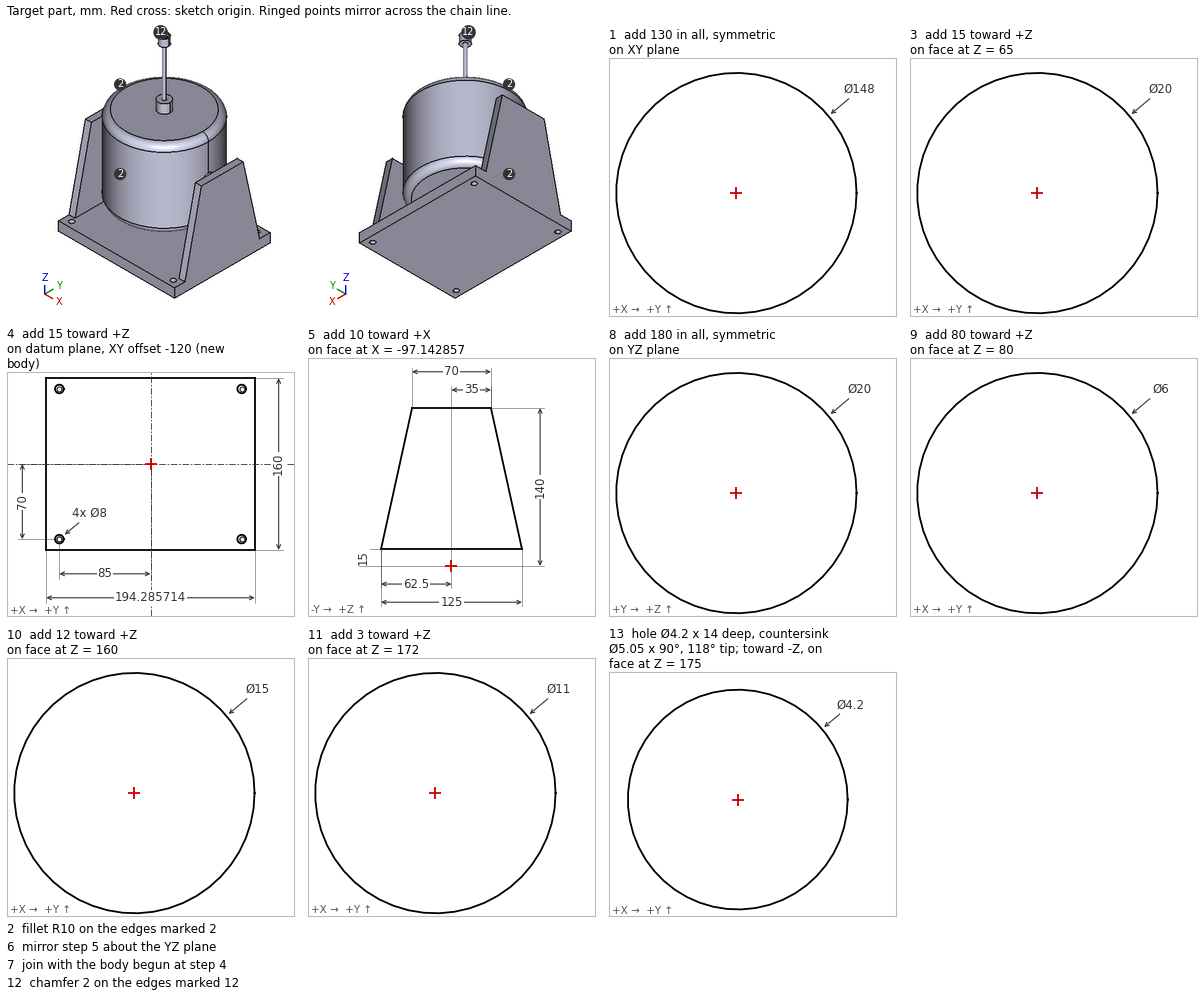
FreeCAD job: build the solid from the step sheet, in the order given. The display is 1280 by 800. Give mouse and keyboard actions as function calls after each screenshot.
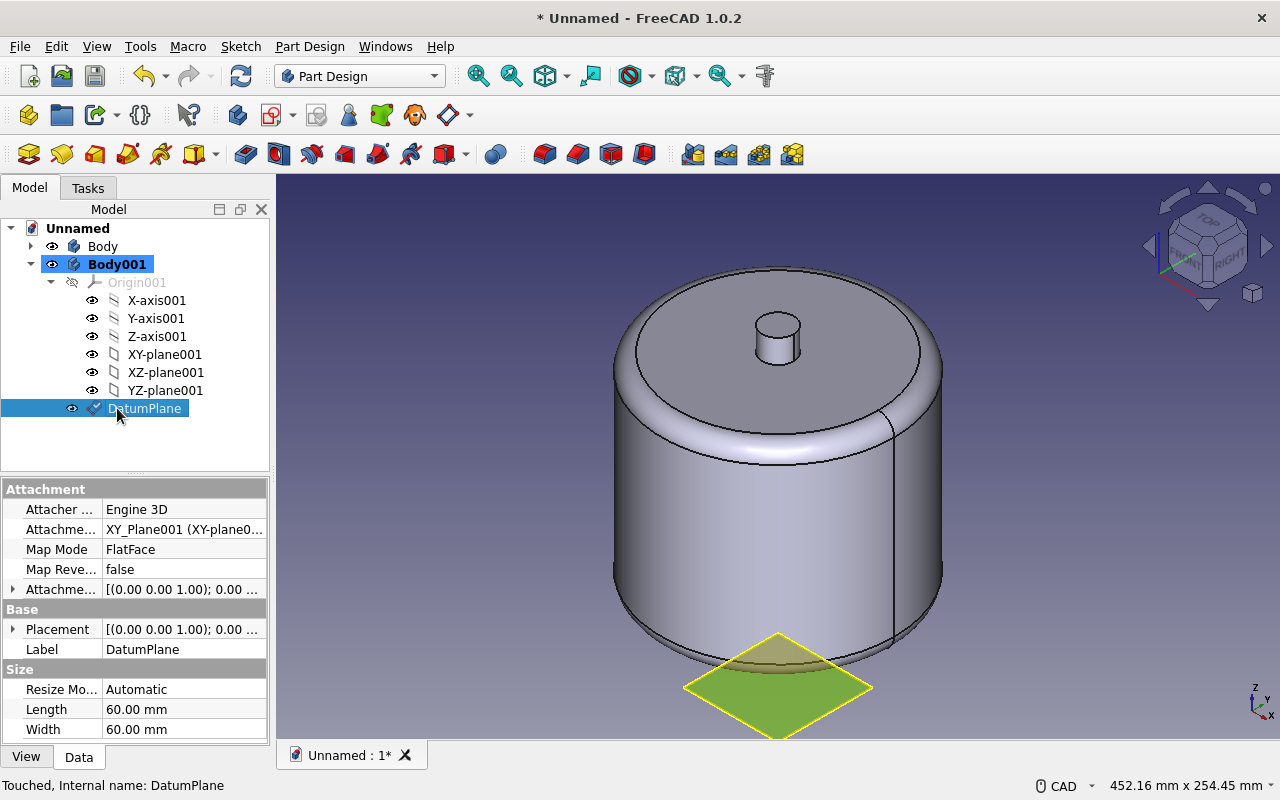
click(270, 116)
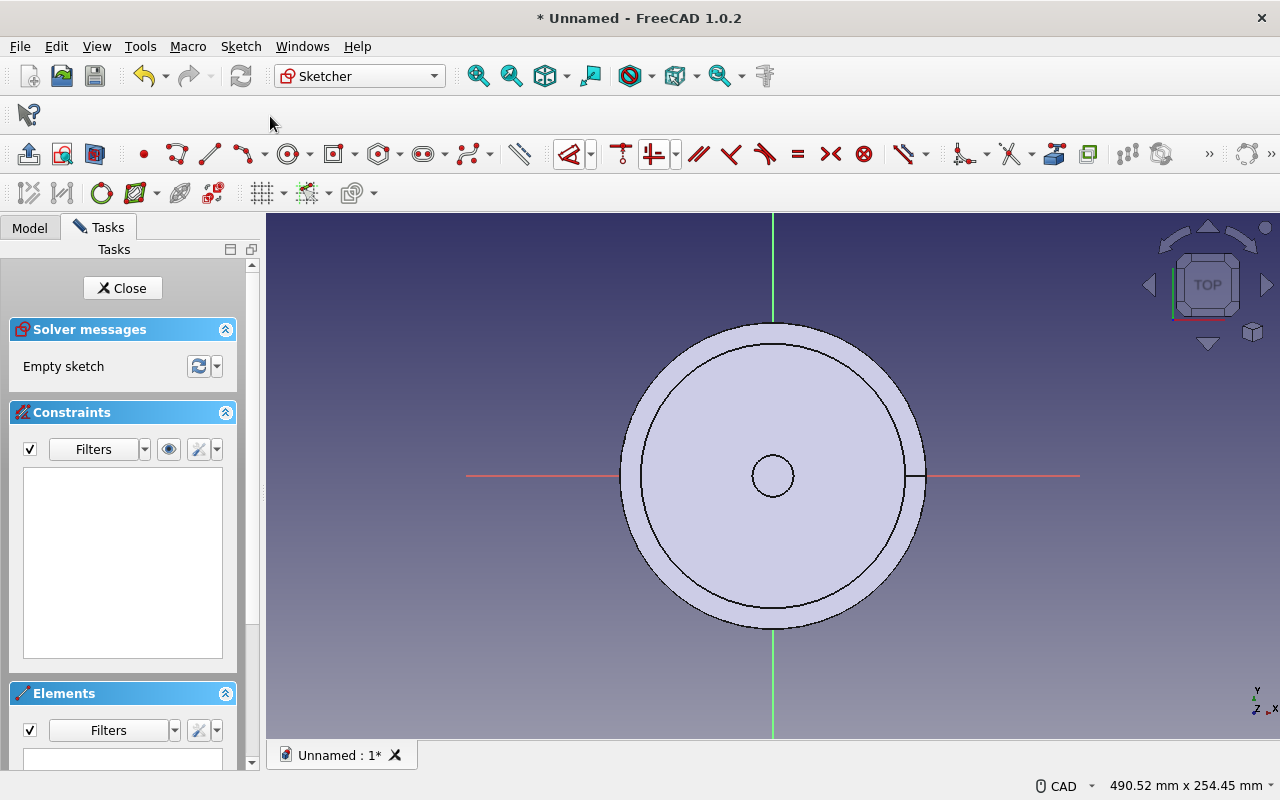
key(g)
key(v)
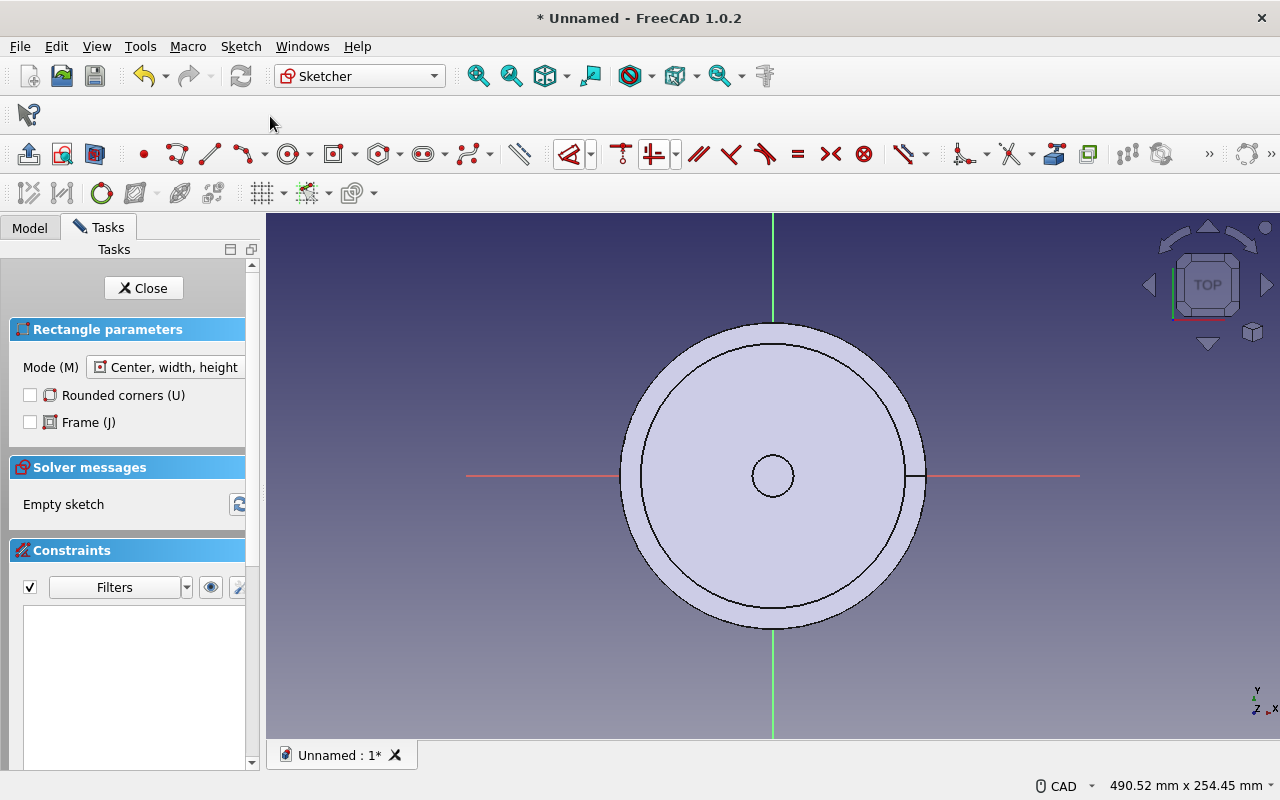
click(773, 476)
click(974, 311)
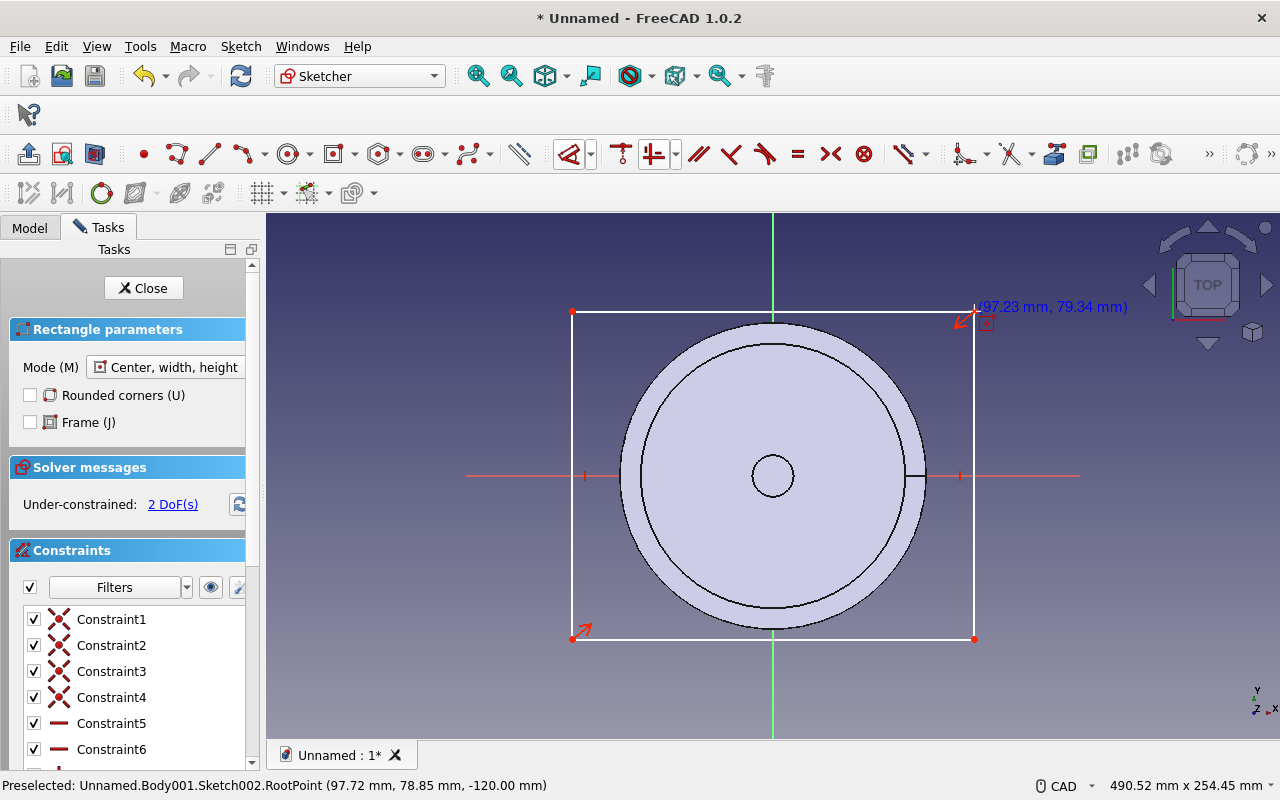
key(g)
key(c)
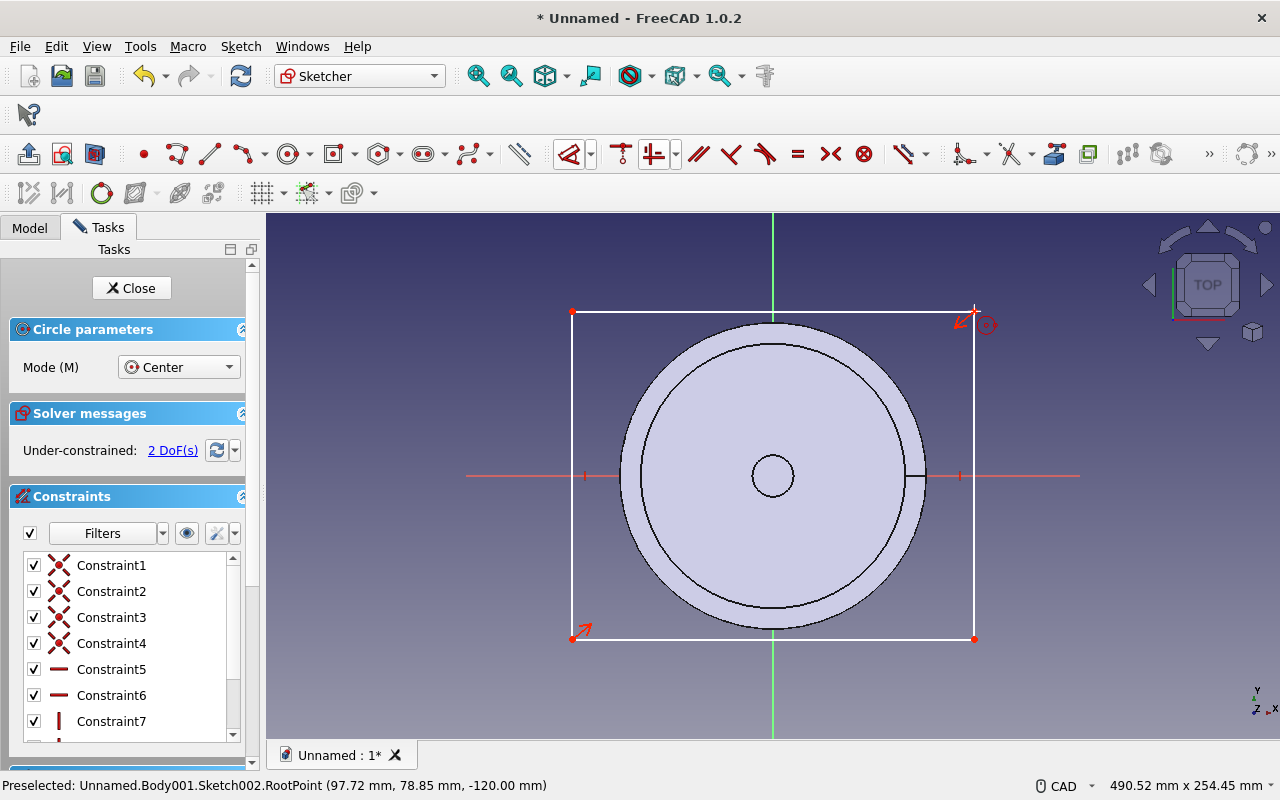
scroll(597, 621, up, 6)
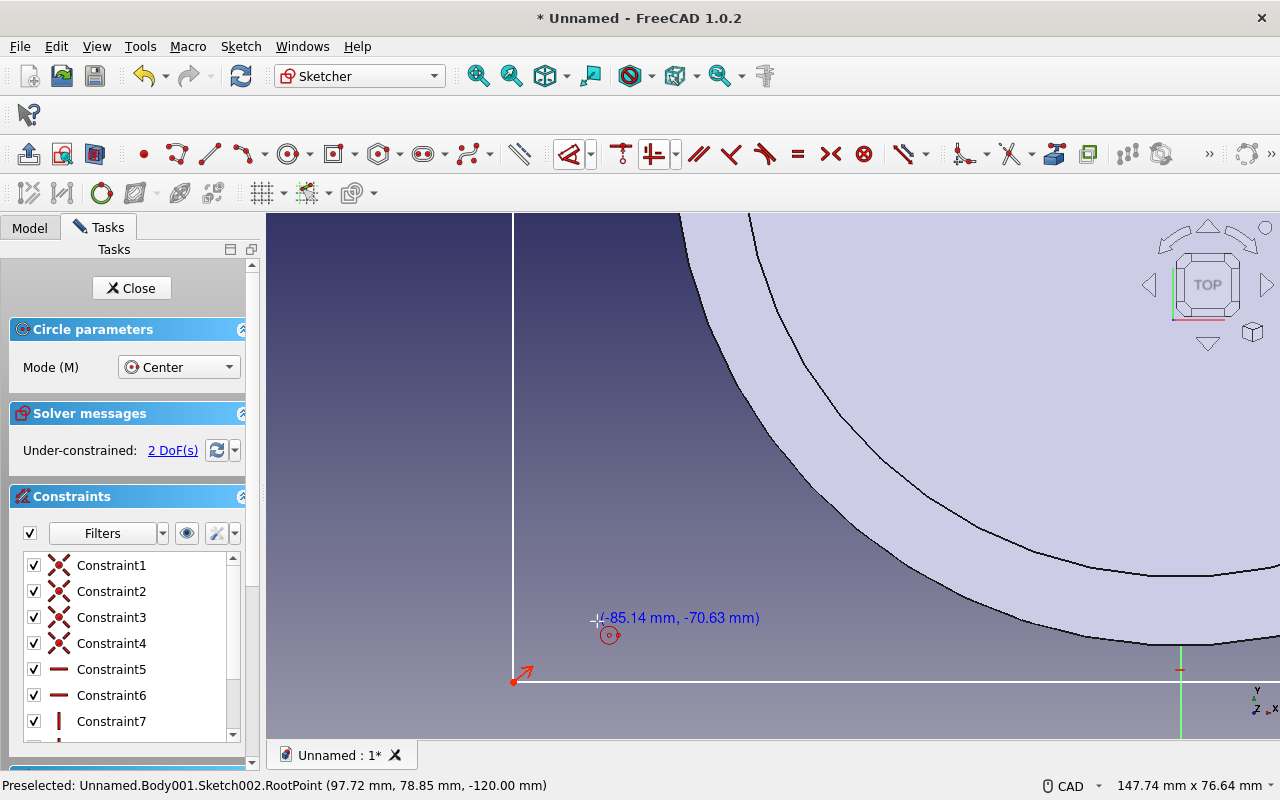
click(597, 618)
click(617, 599)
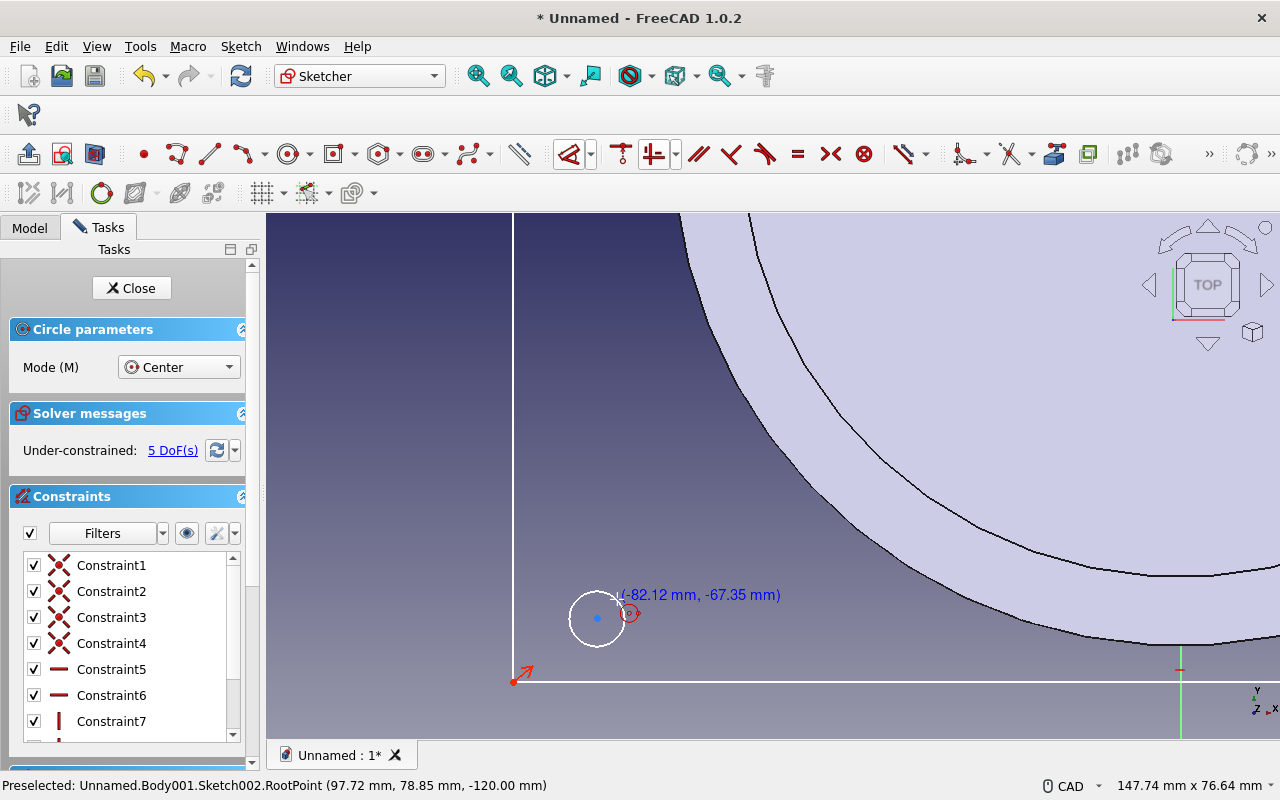
scroll(499, 622, down, 6)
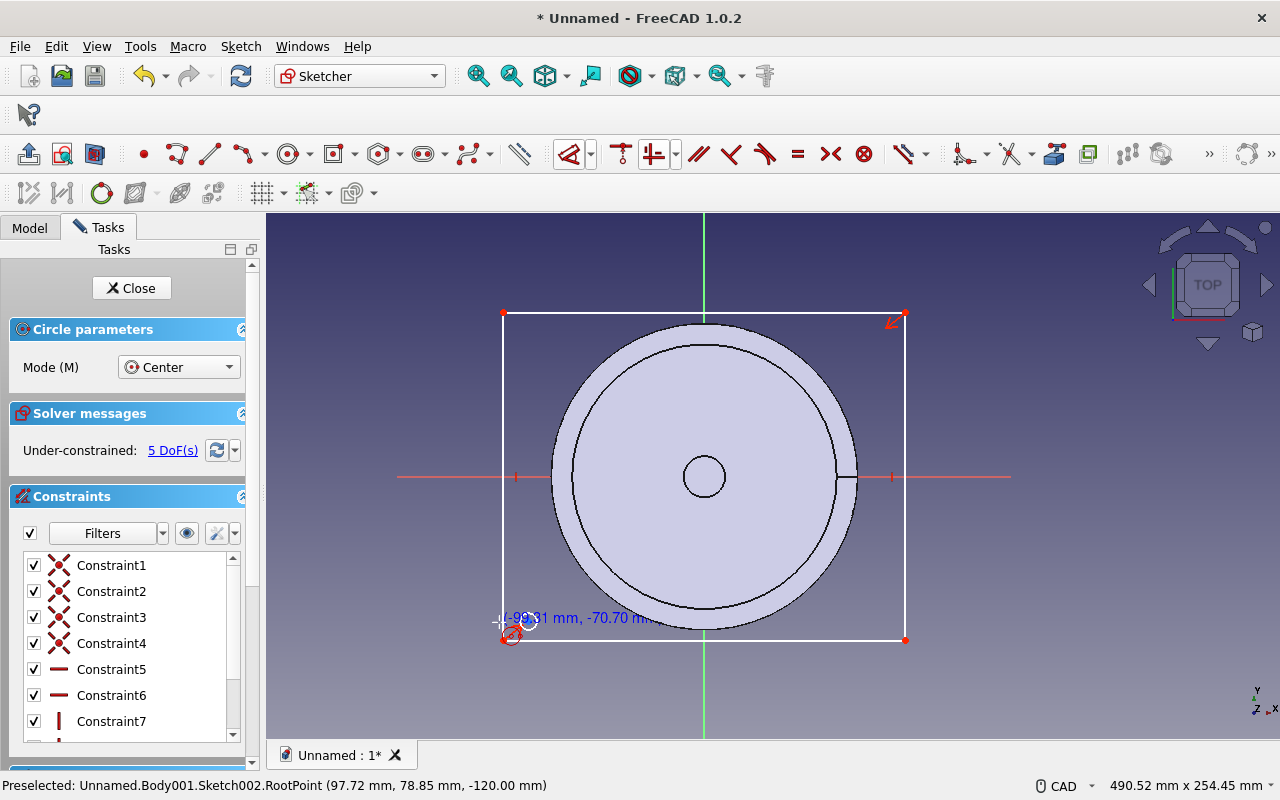
scroll(880, 621, up, 6)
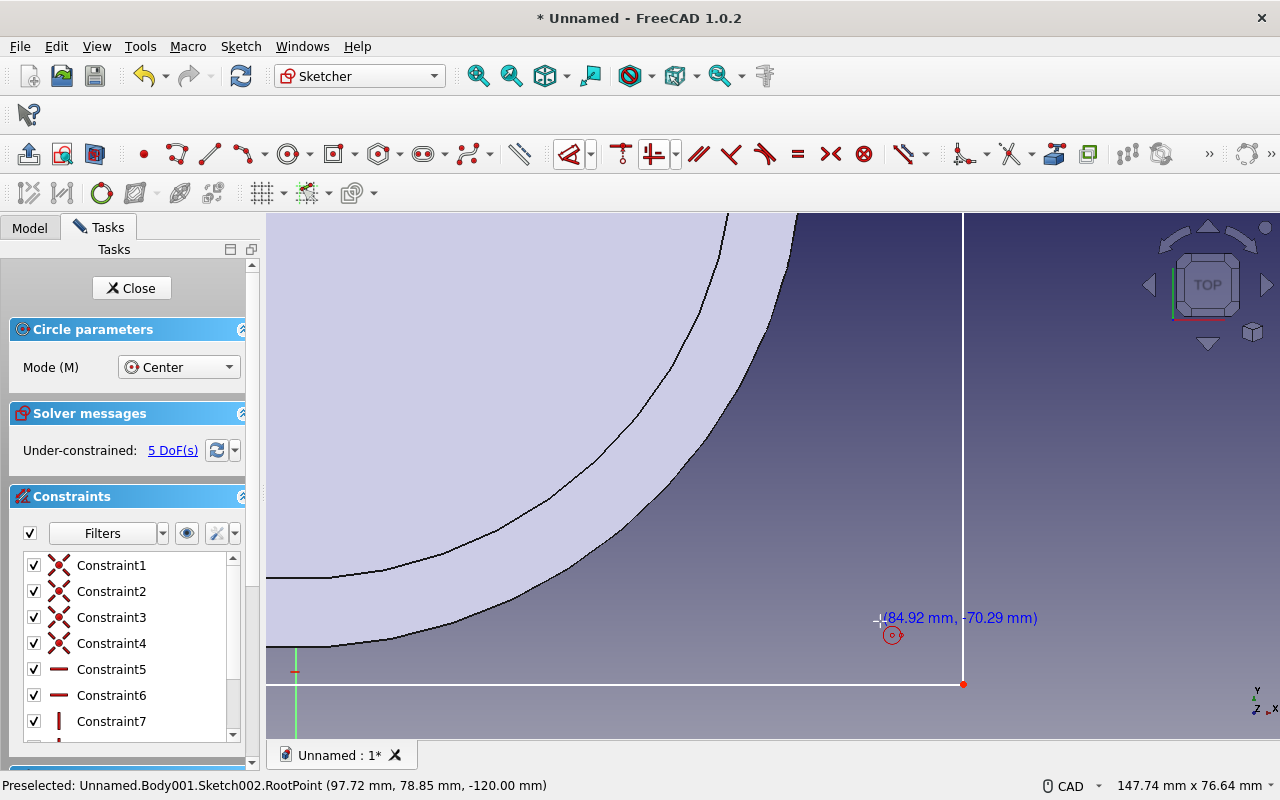
click(879, 621)
click(899, 601)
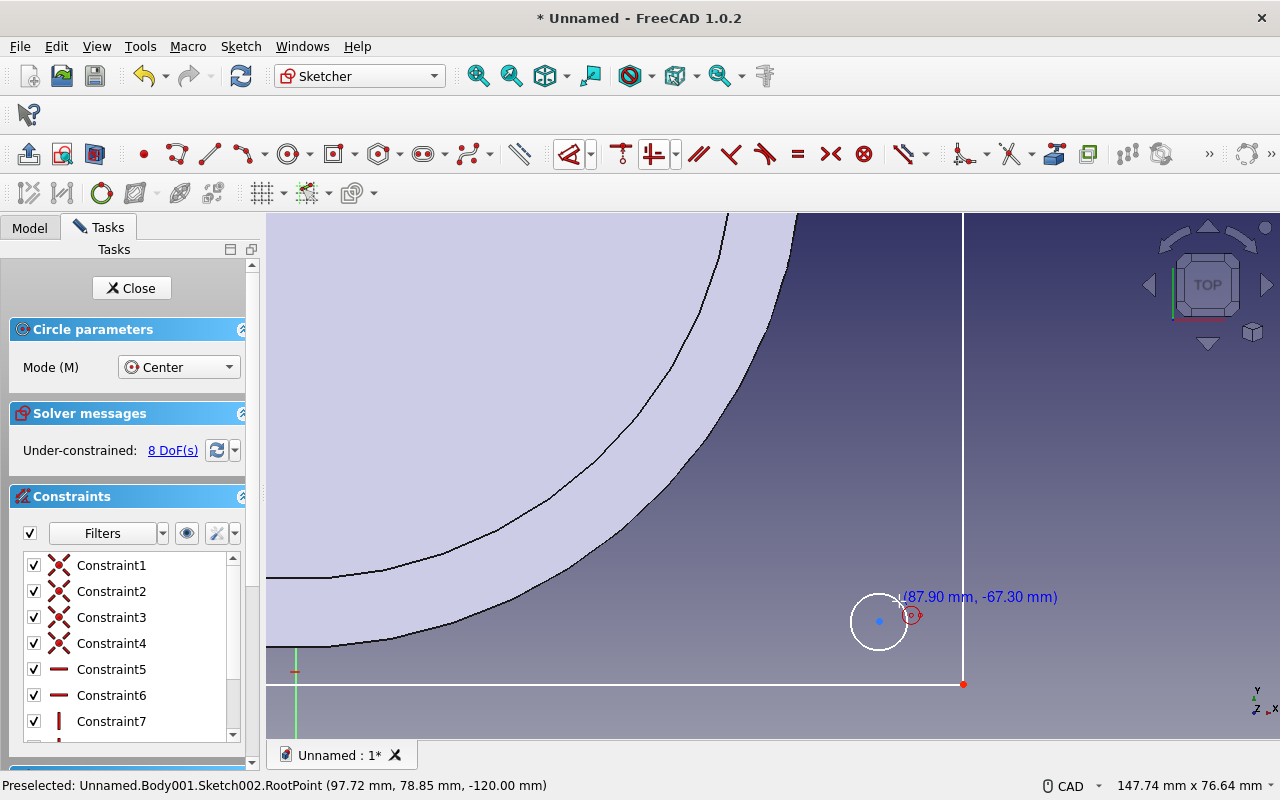
scroll(881, 621, down, 6)